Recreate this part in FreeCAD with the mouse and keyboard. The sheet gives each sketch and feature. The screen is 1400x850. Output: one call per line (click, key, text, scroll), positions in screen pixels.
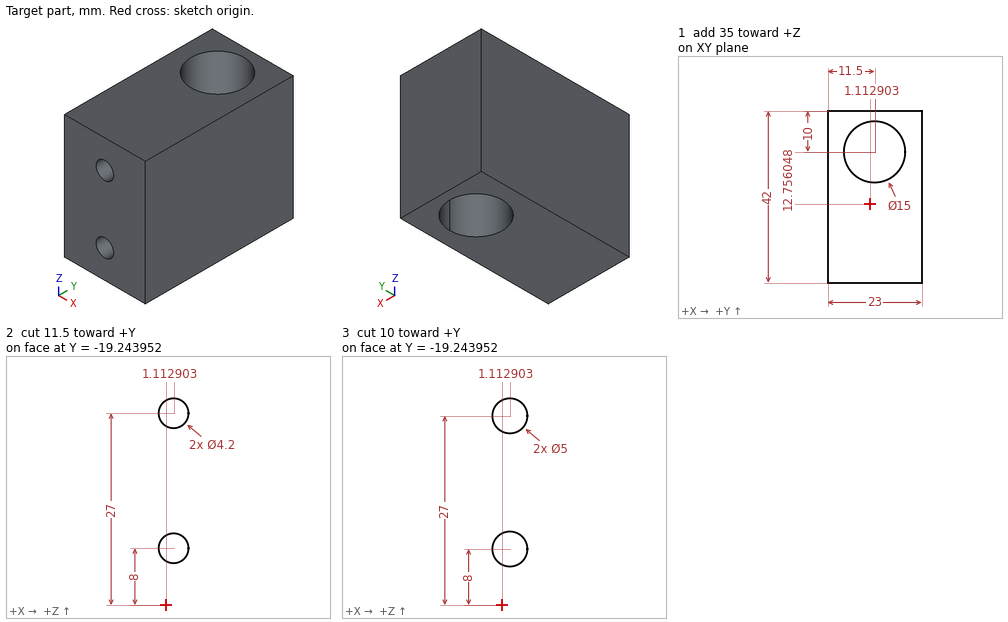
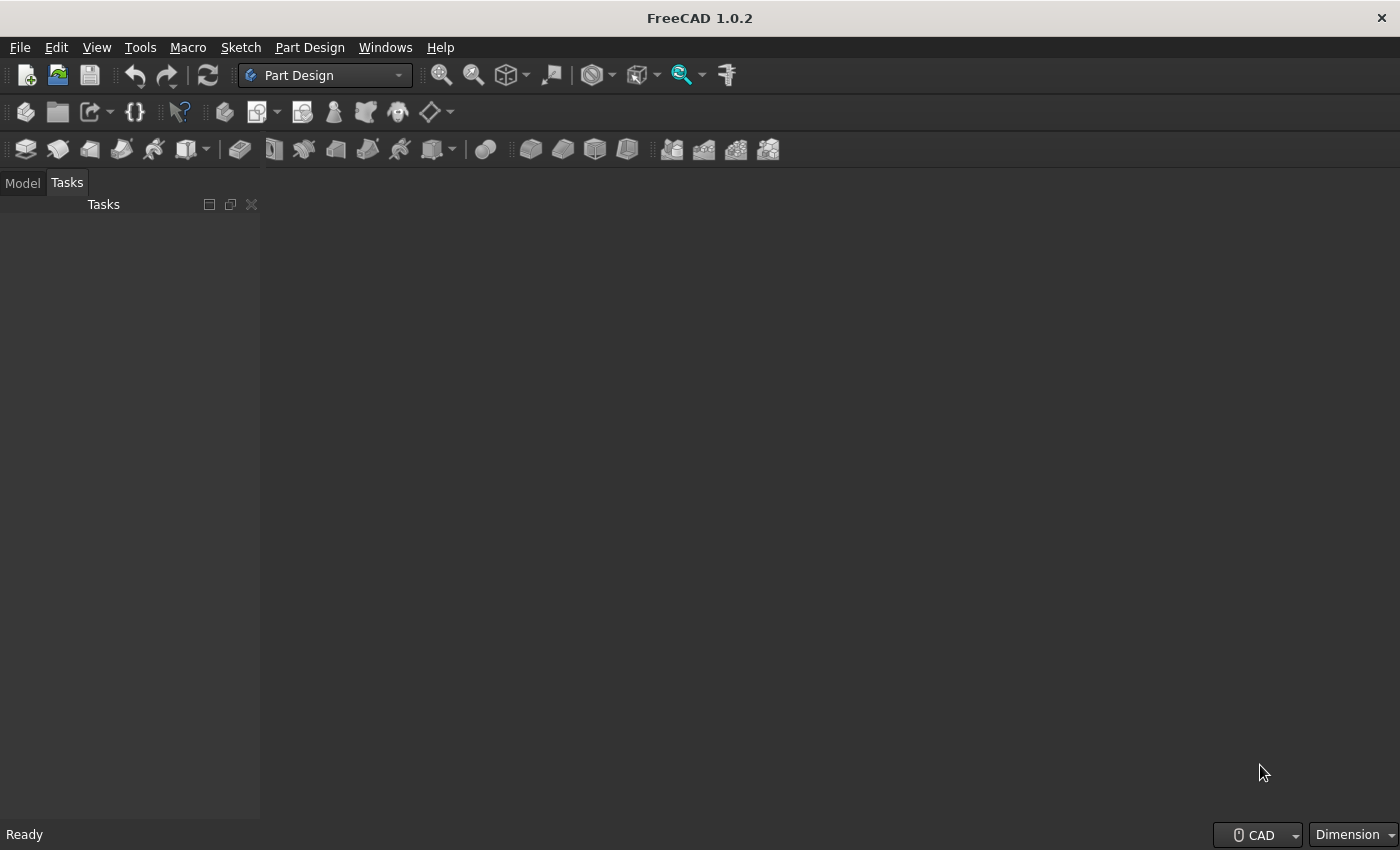
click(26, 76)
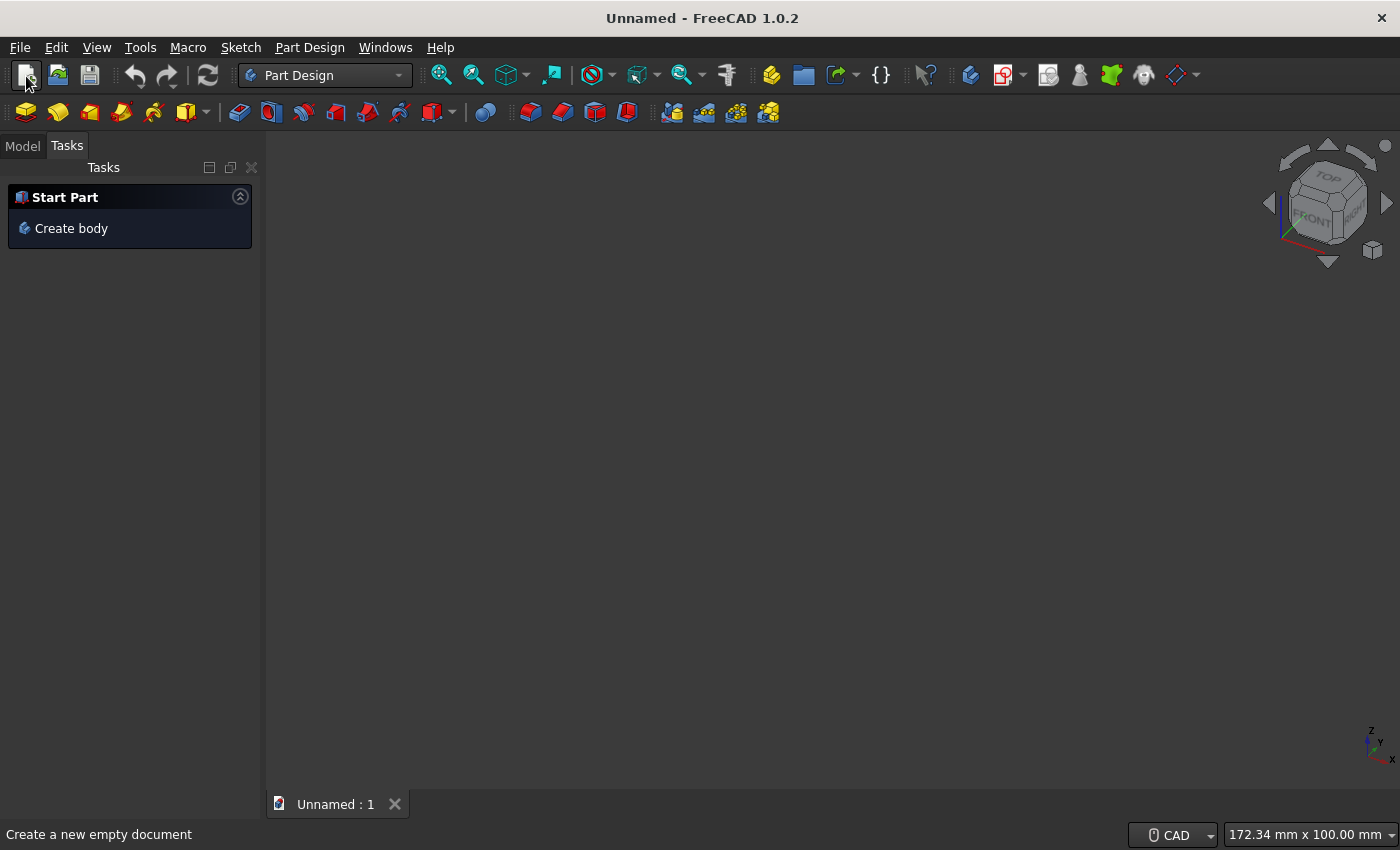
click(1004, 76)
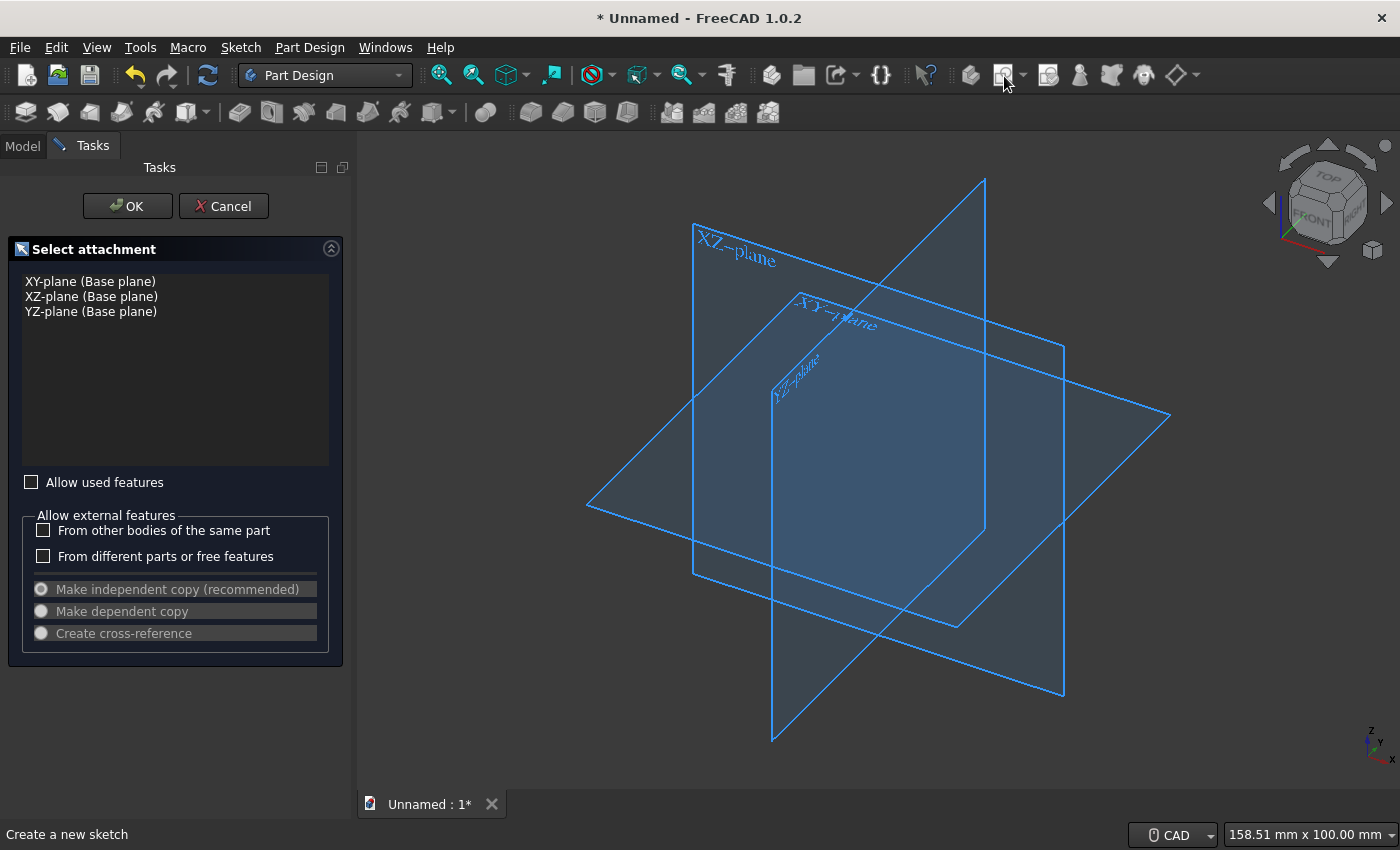
click(82, 282)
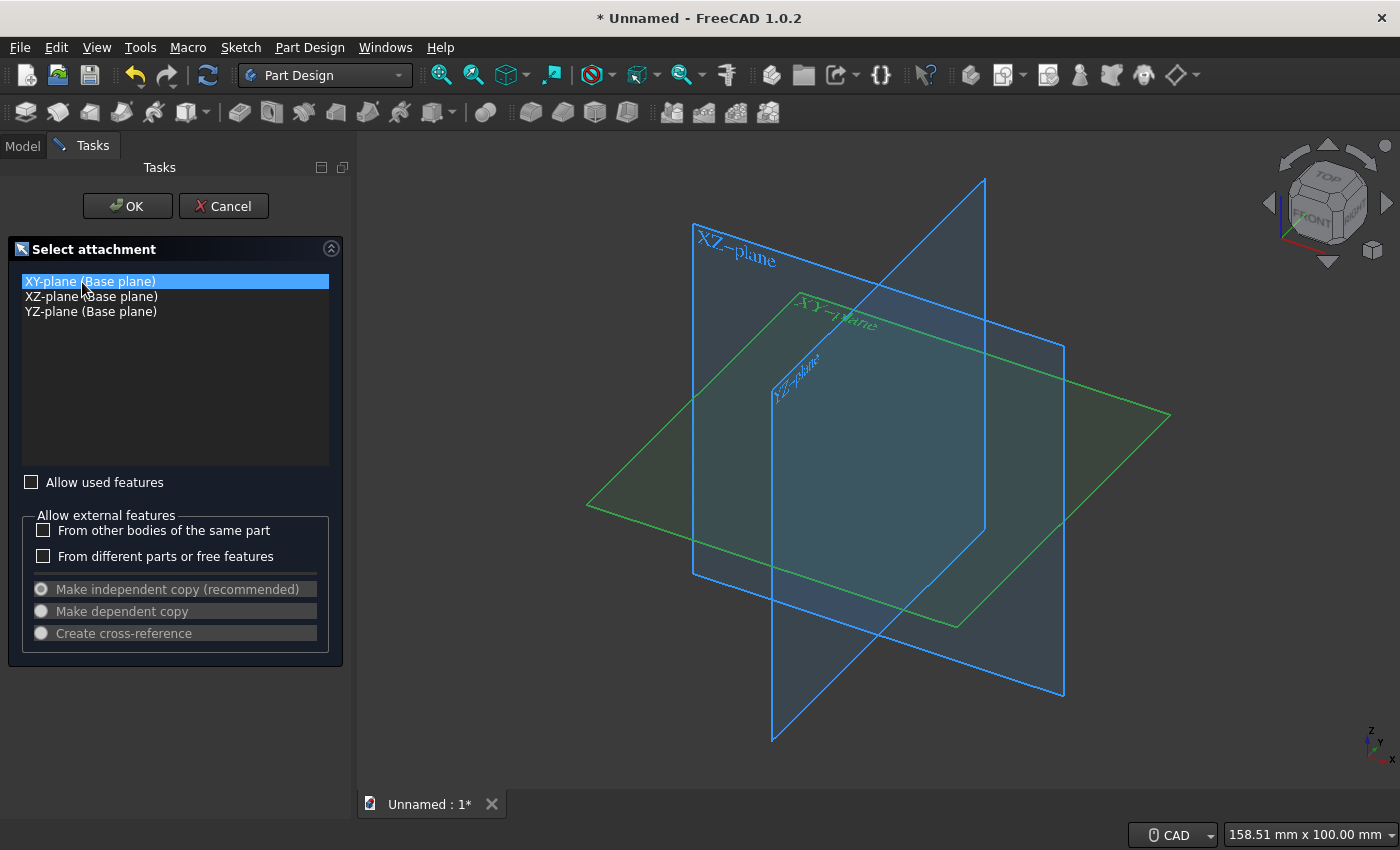
click(128, 206)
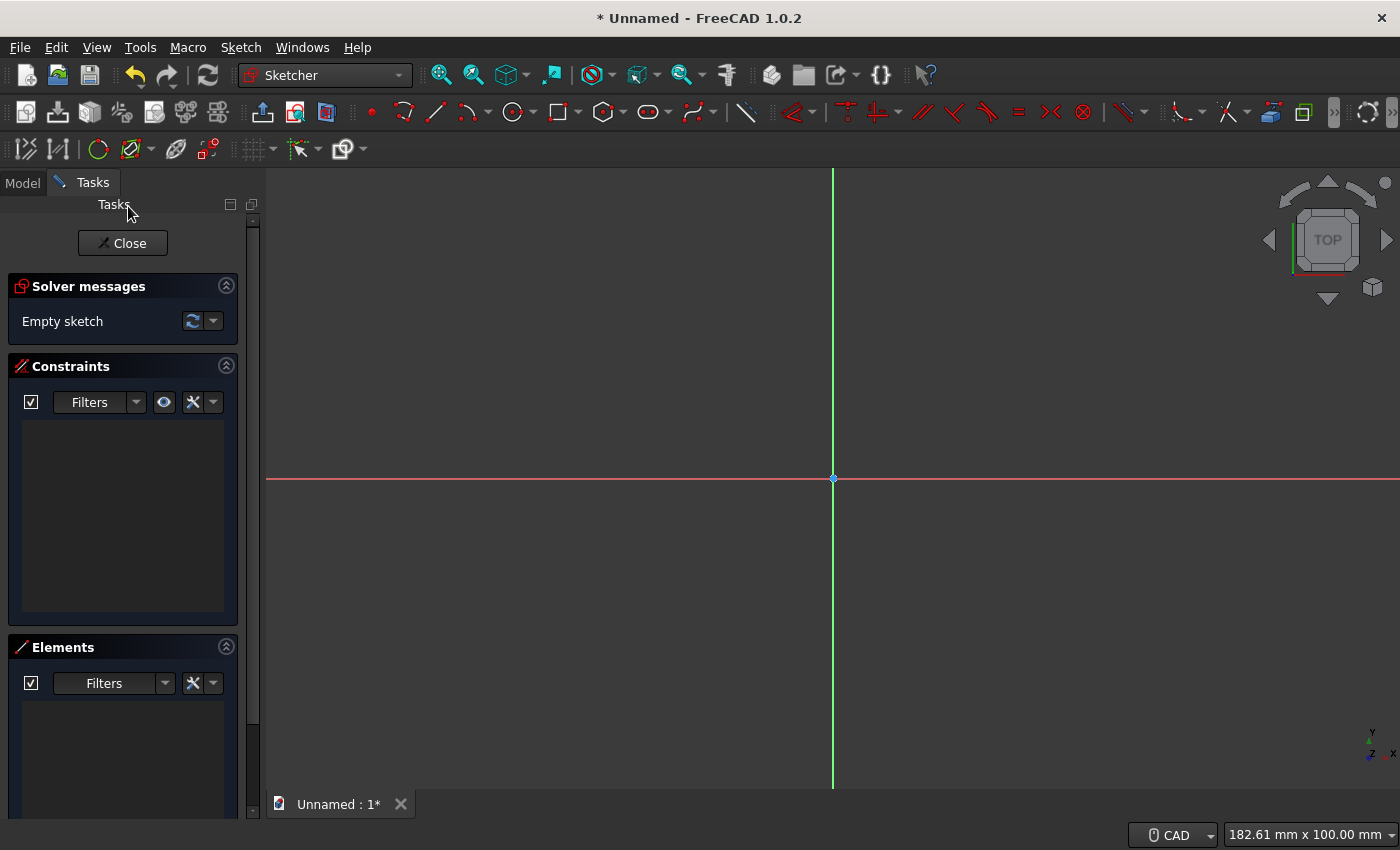
scroll(993, 445, up, 2)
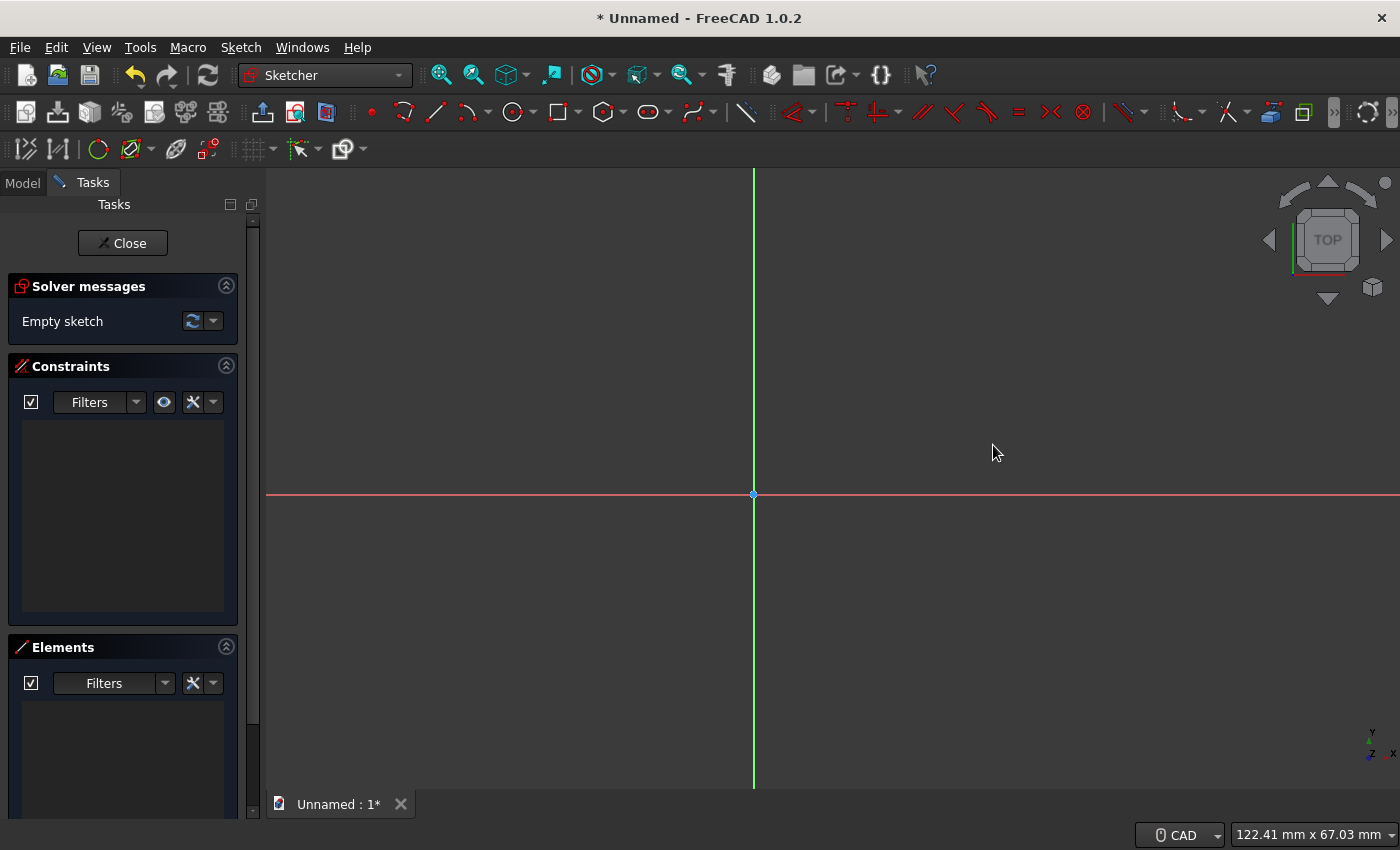
click(558, 112)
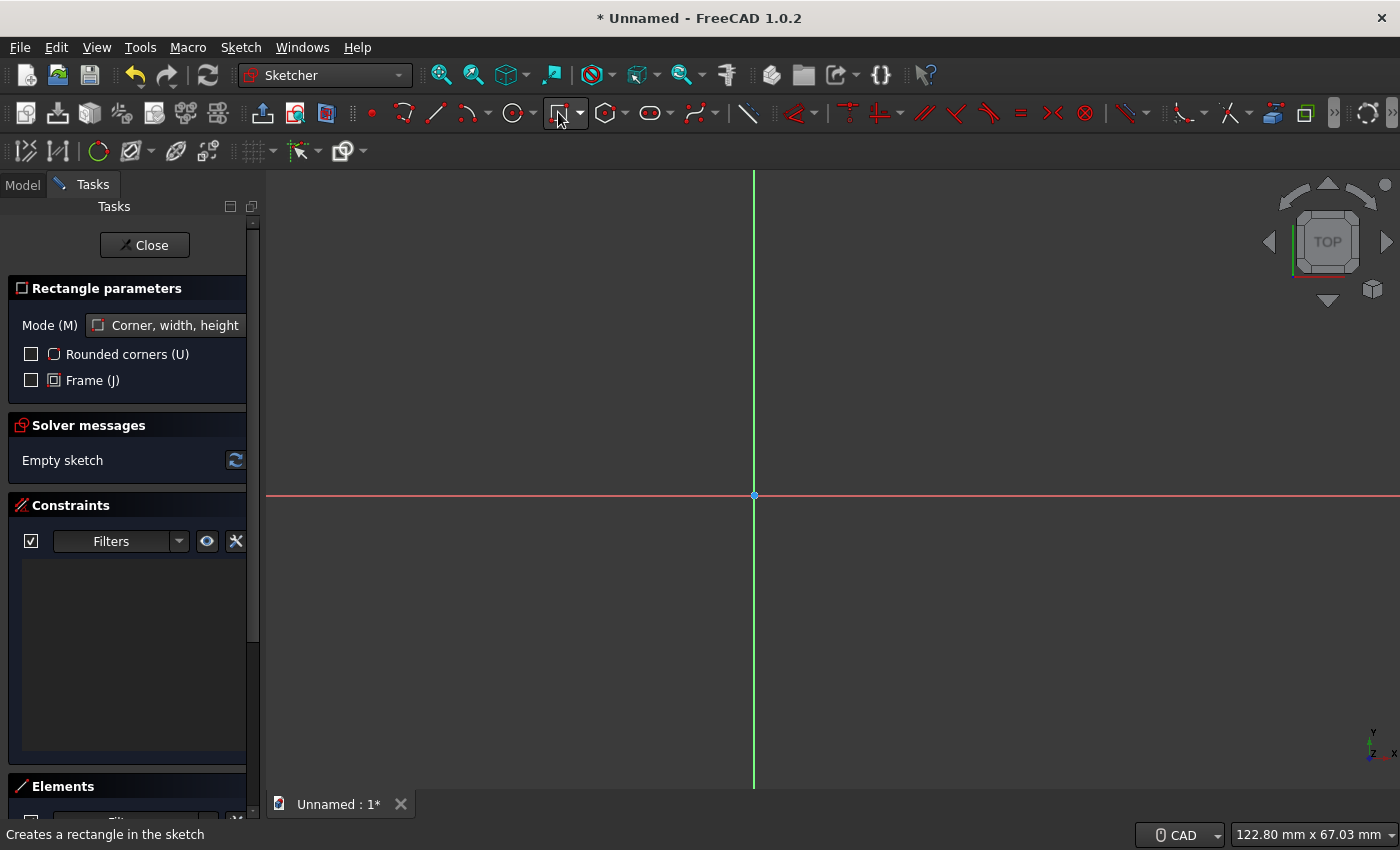
click(658, 286)
click(871, 673)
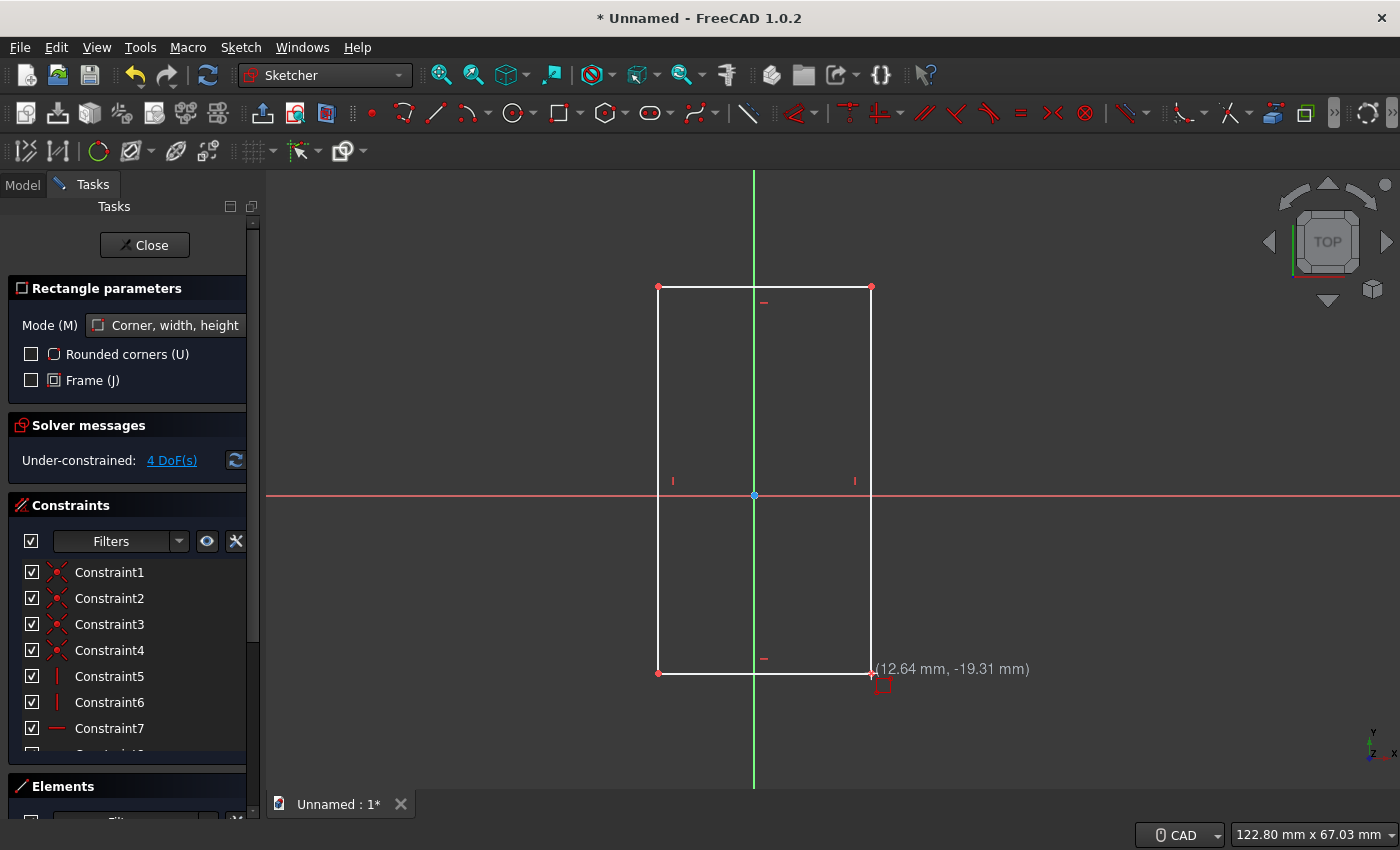
click(514, 114)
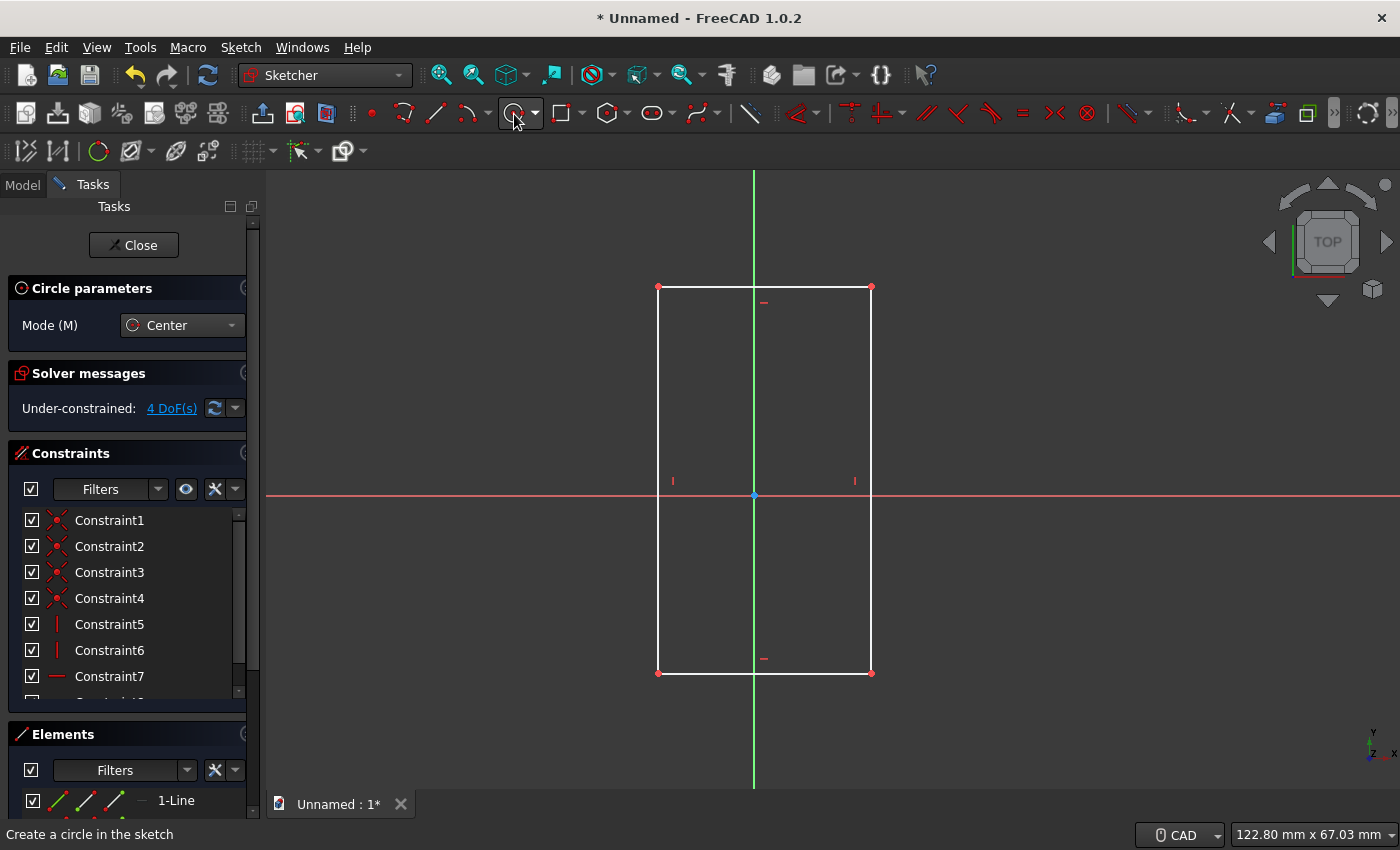
scroll(765, 378, up, 3)